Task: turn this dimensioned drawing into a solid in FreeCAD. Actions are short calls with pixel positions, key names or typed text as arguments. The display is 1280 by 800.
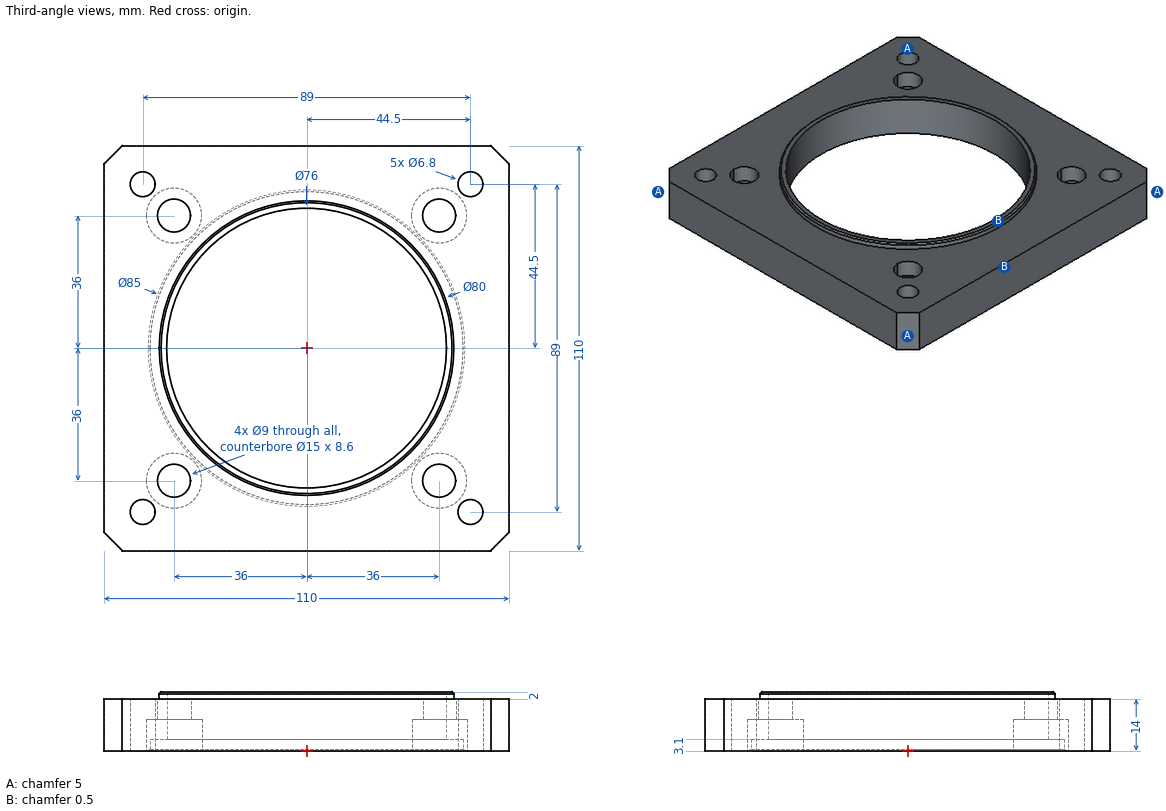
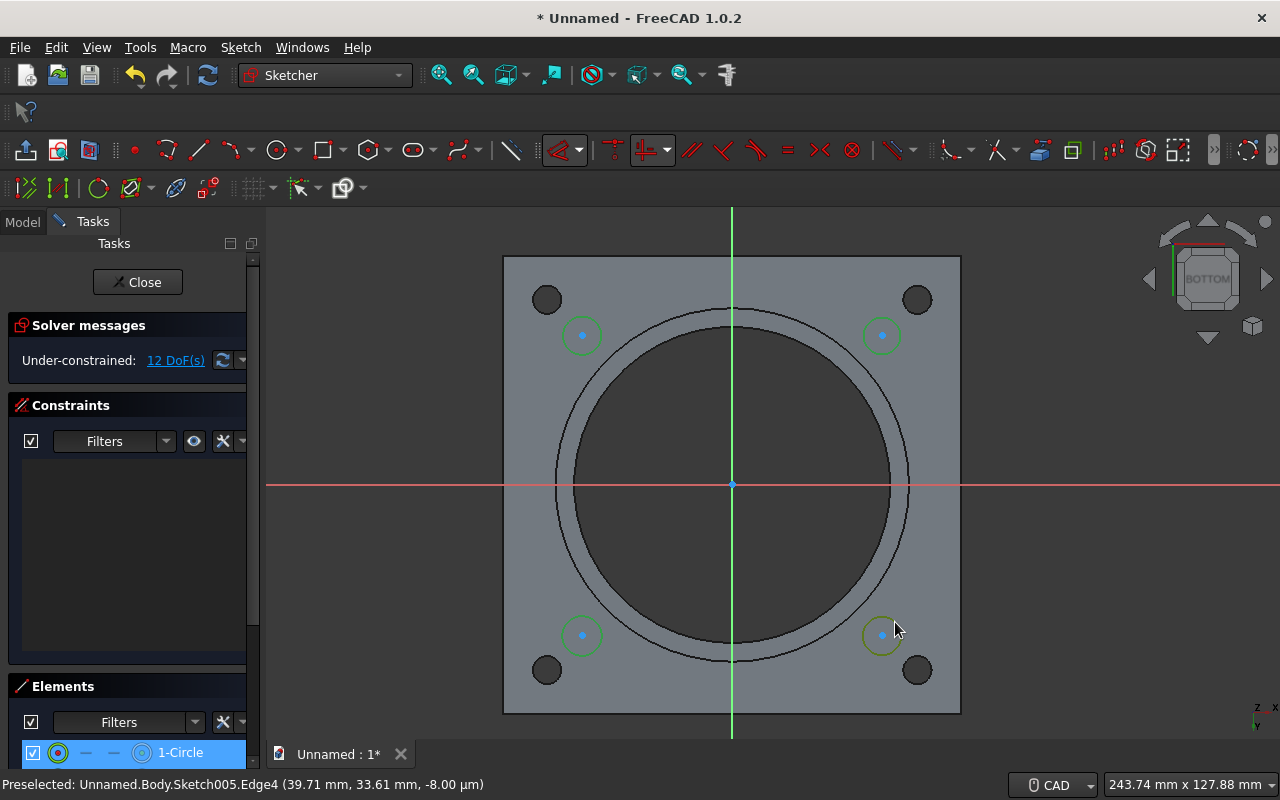
click(788, 150)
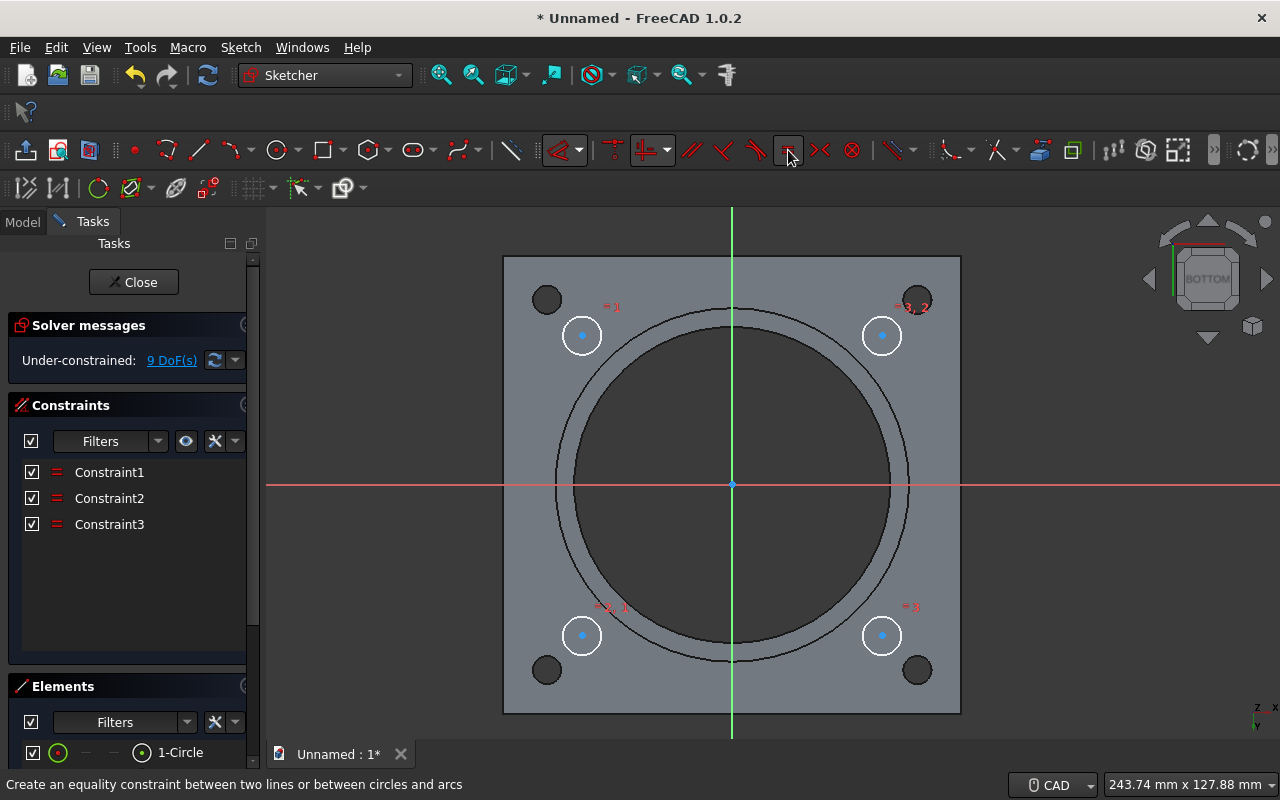
click(582, 336)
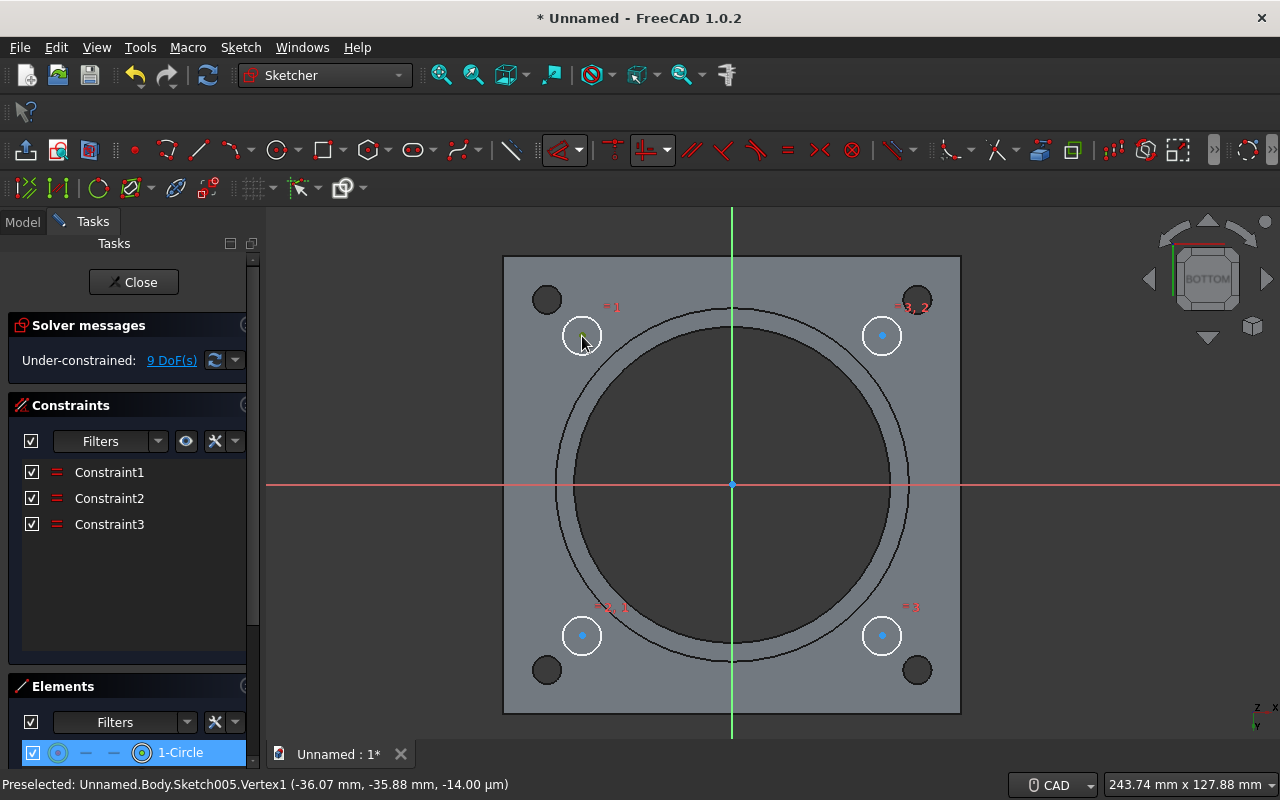
click(582, 636)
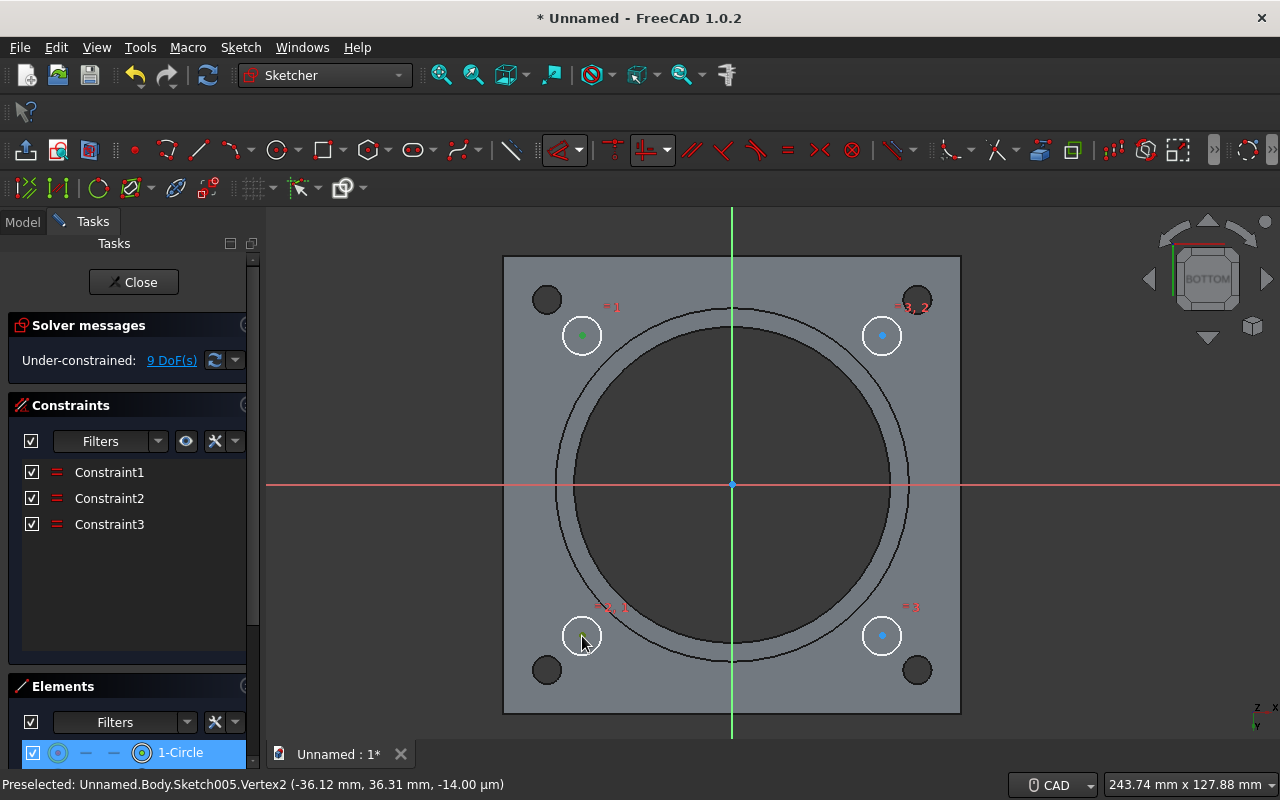
click(670, 150)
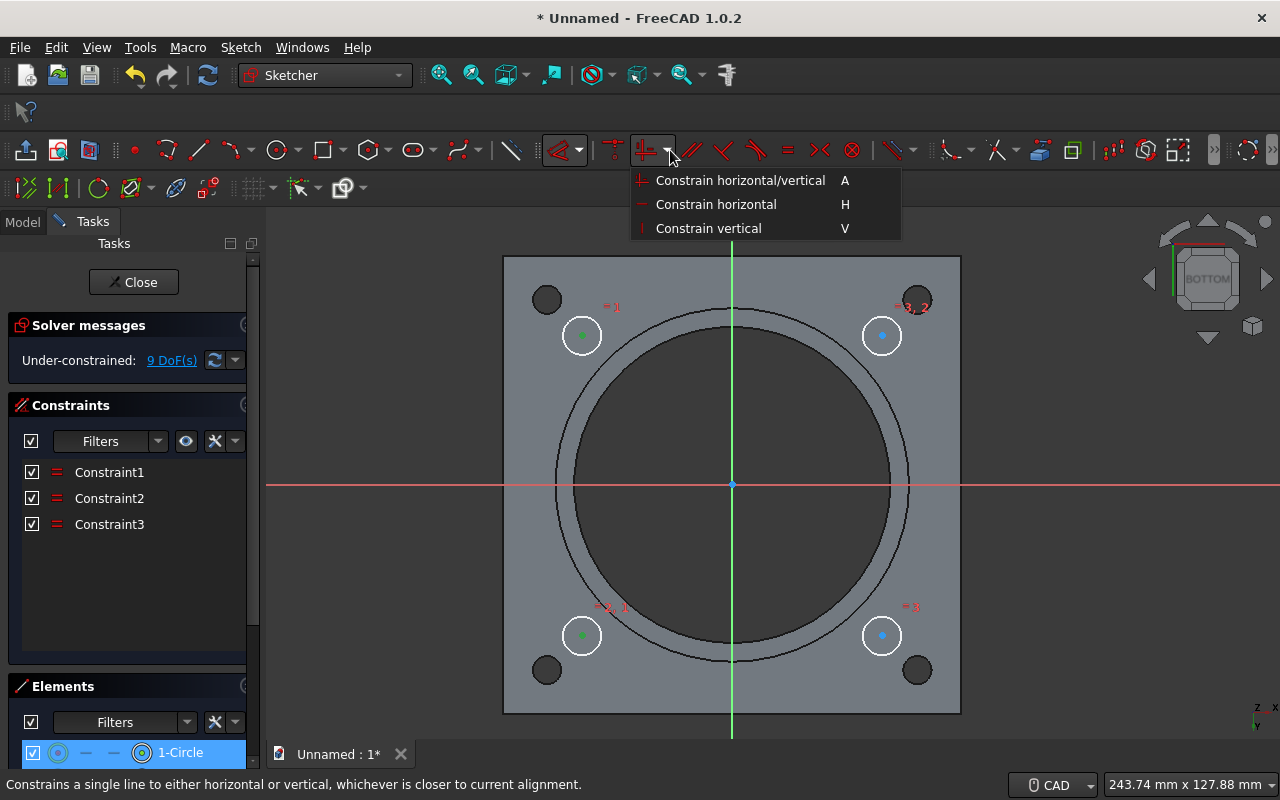
click(766, 228)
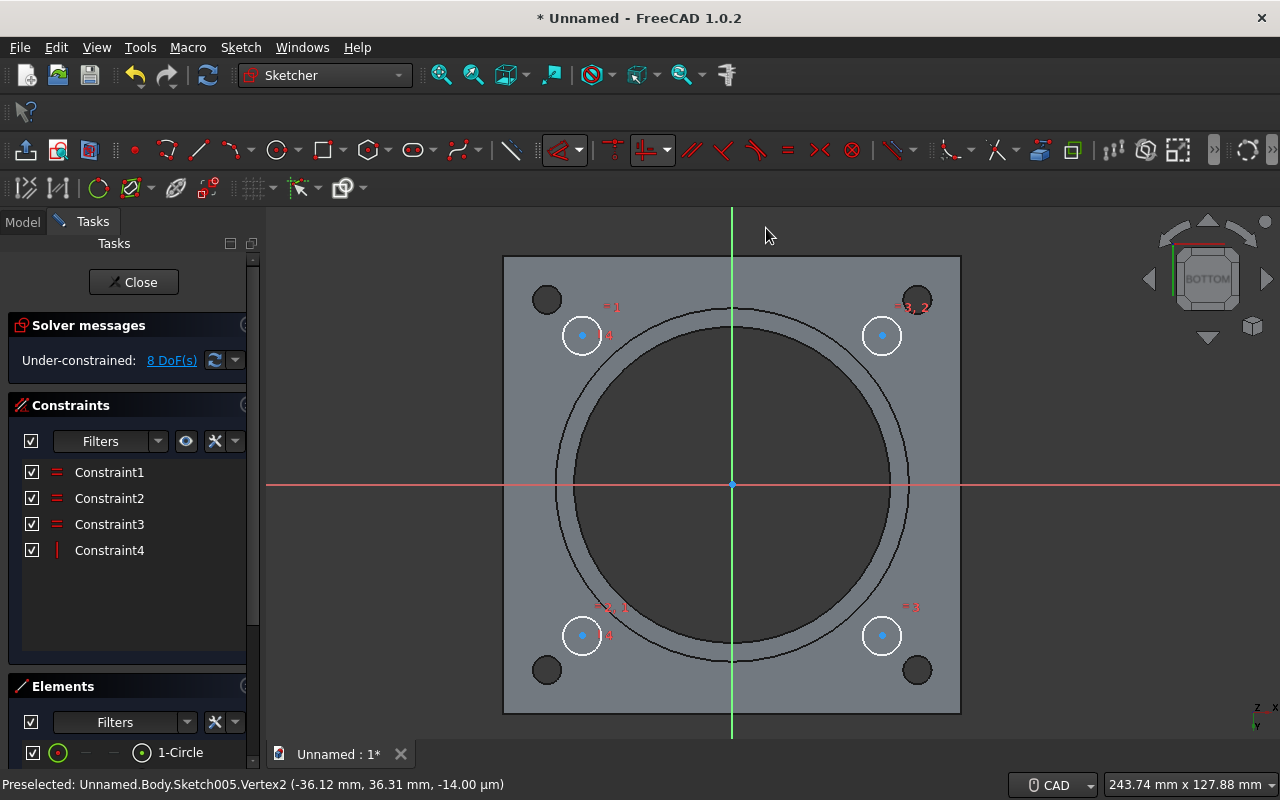
click(582, 336)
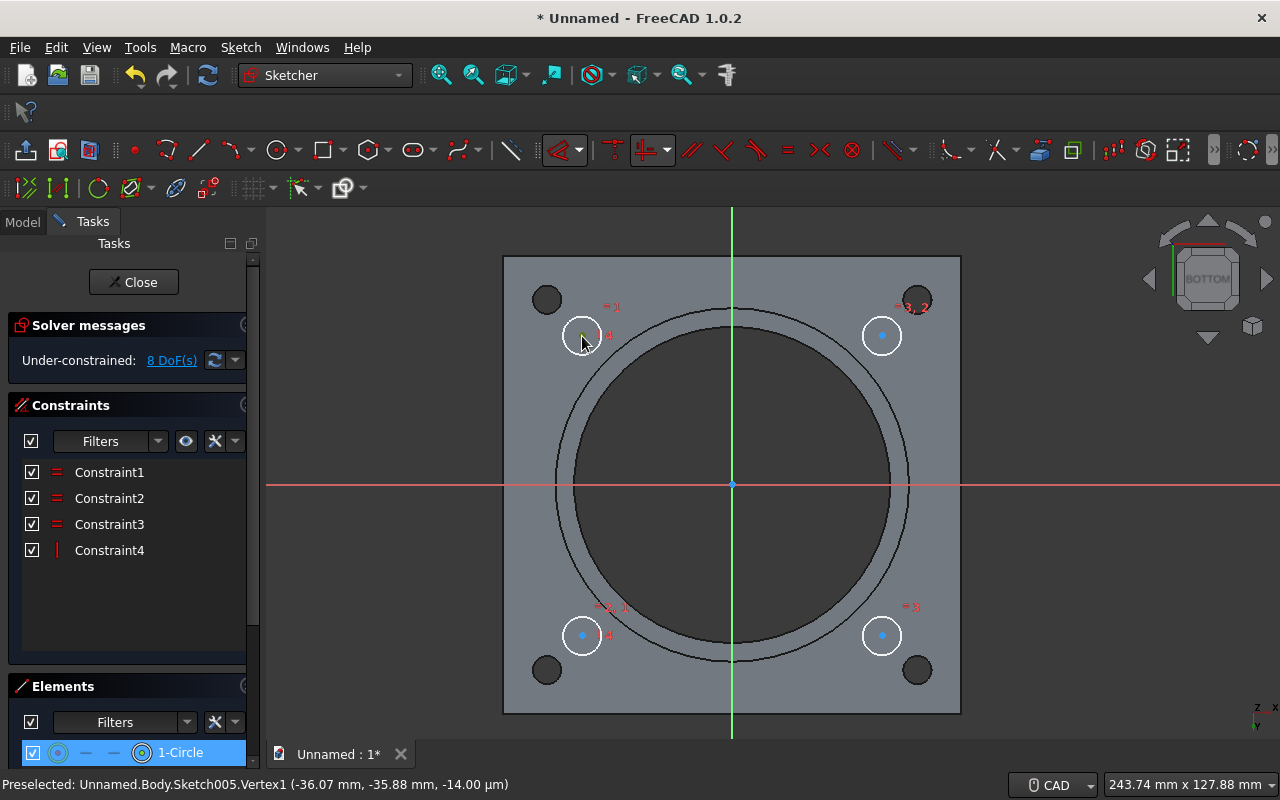
click(882, 336)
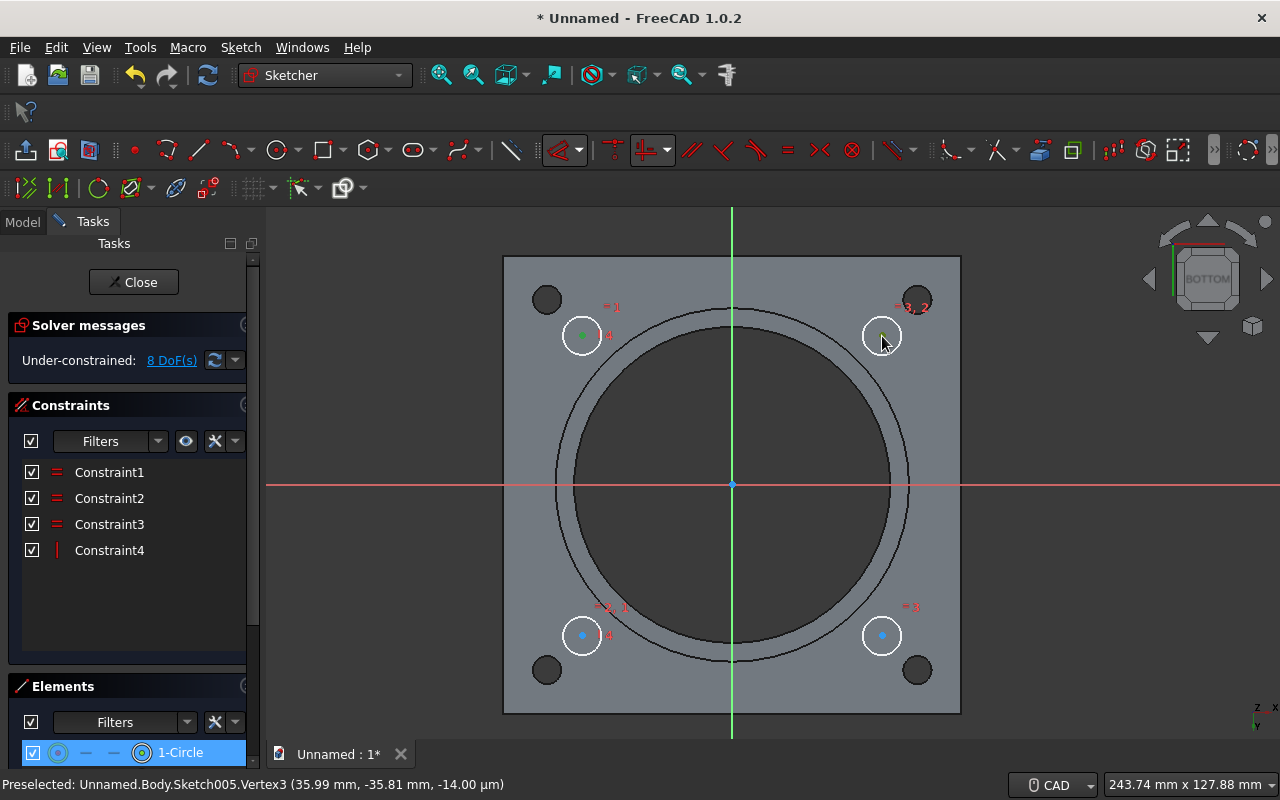
key(h)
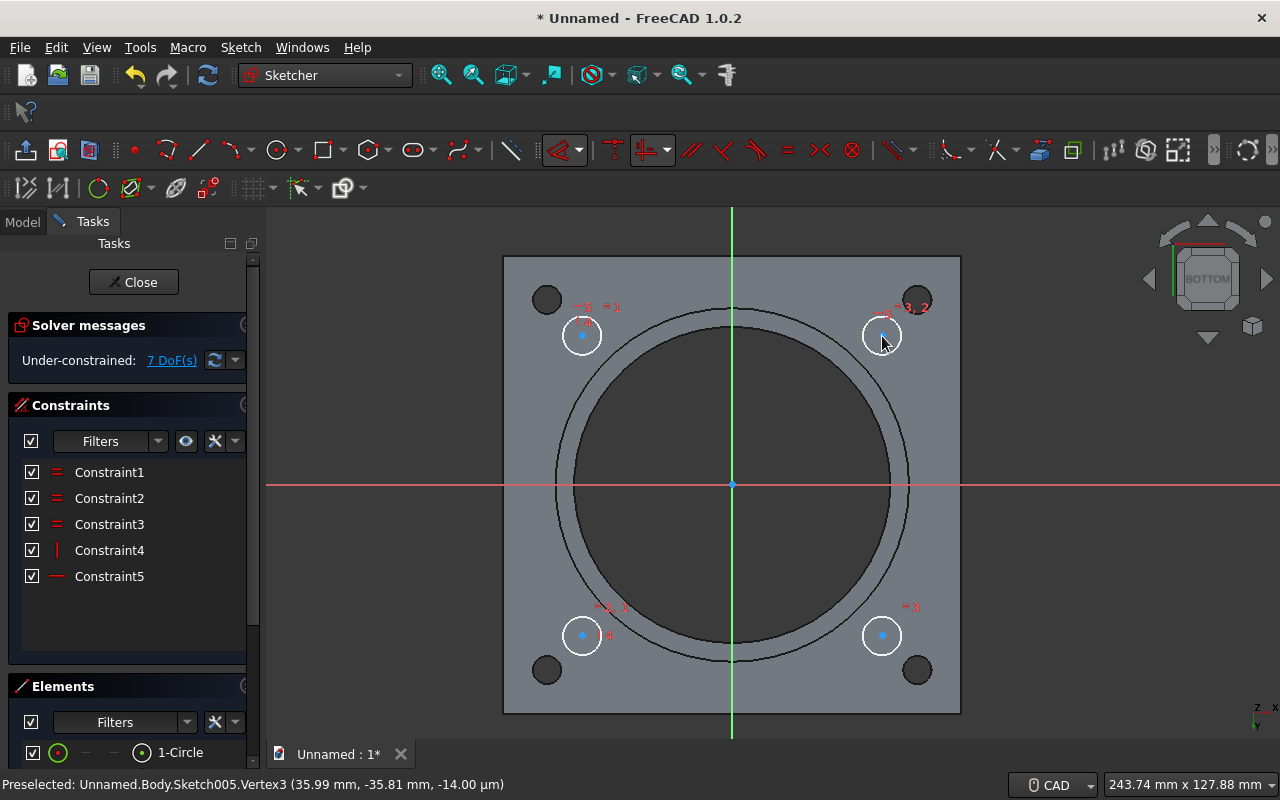
click(882, 336)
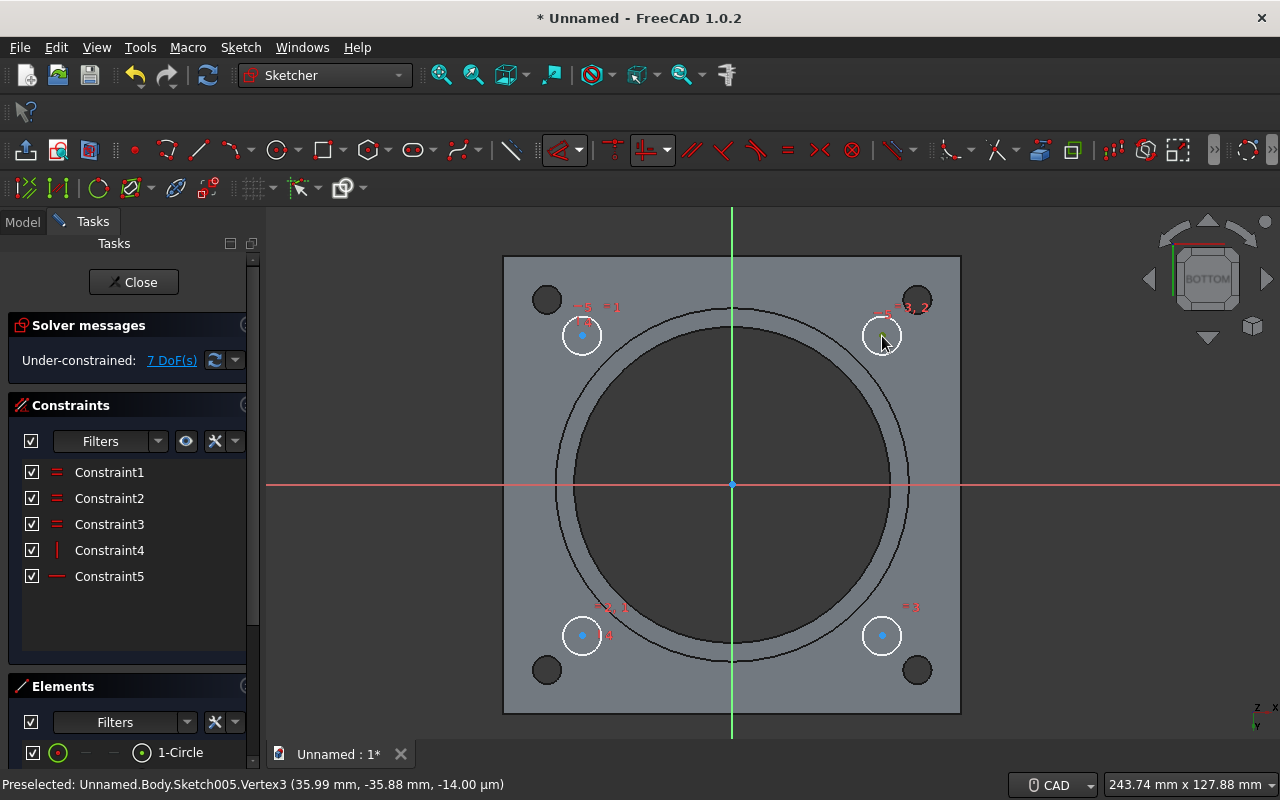
click(882, 636)